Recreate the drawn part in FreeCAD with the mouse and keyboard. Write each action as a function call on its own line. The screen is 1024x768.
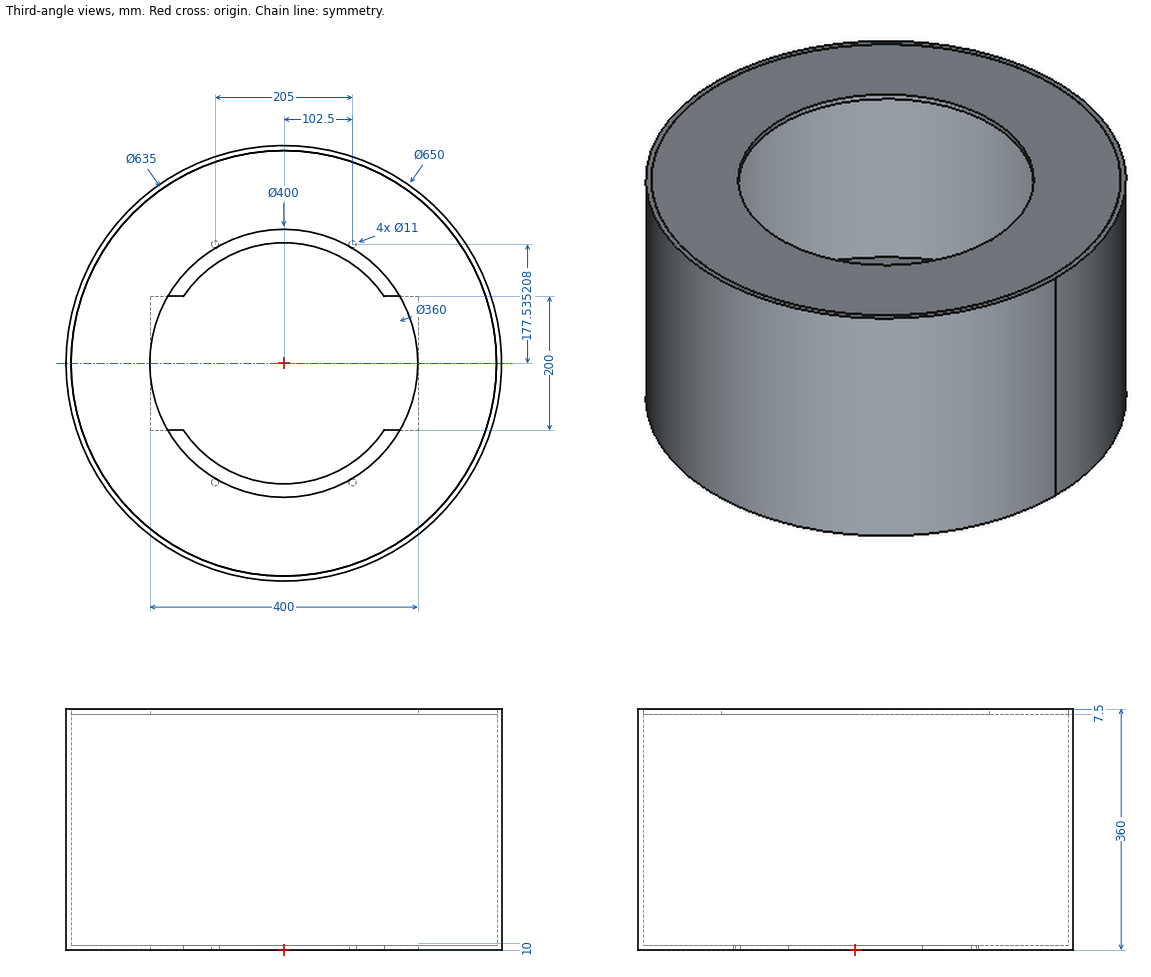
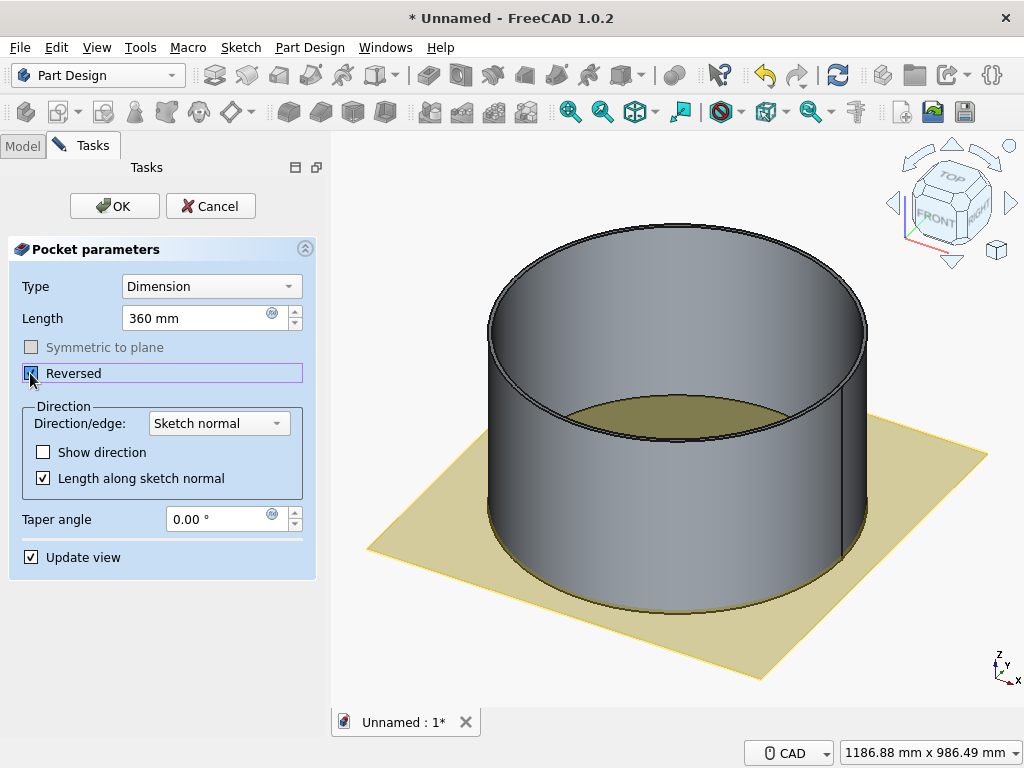
click(115, 206)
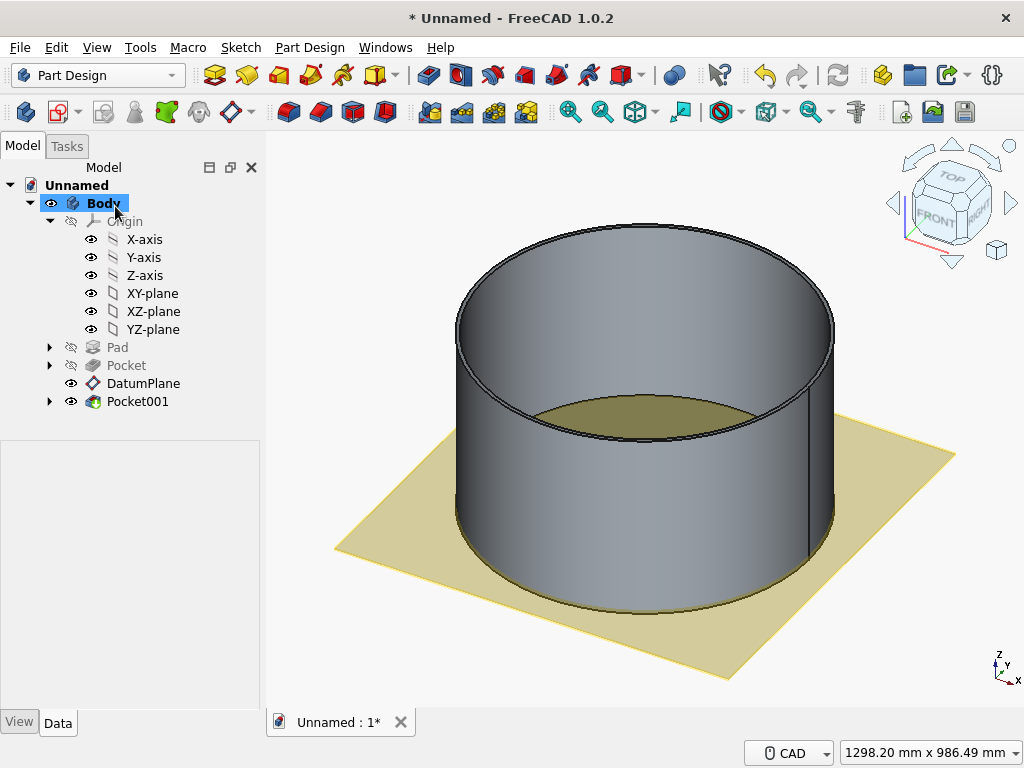
click(116, 383)
key(space)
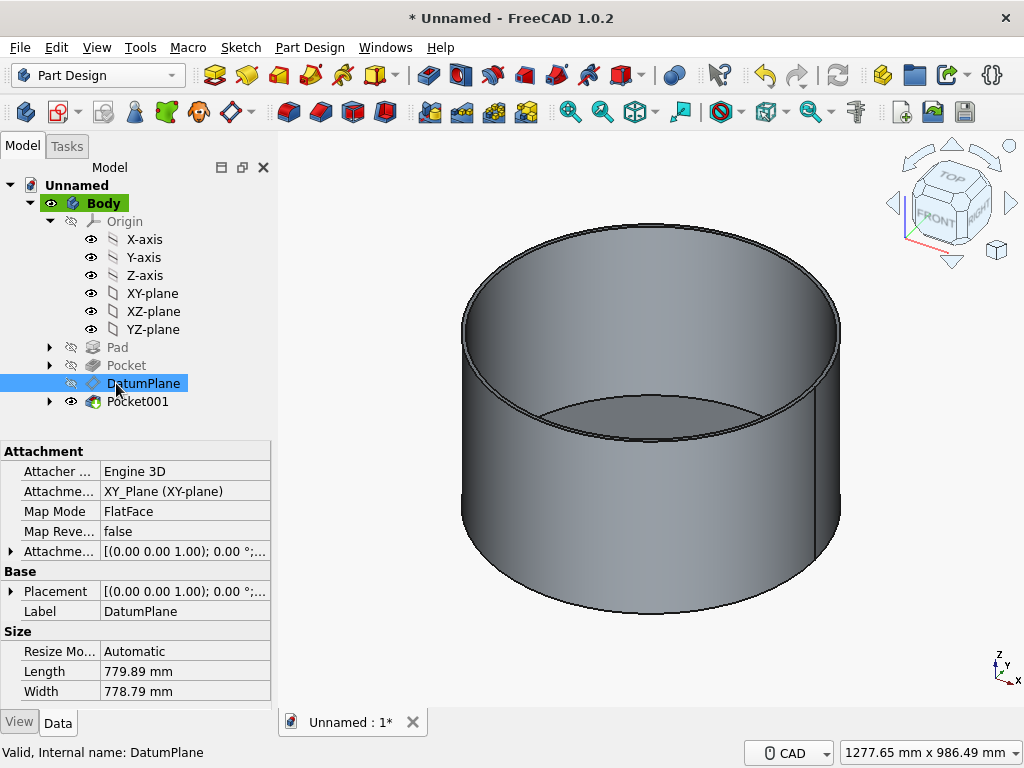
click(318, 667)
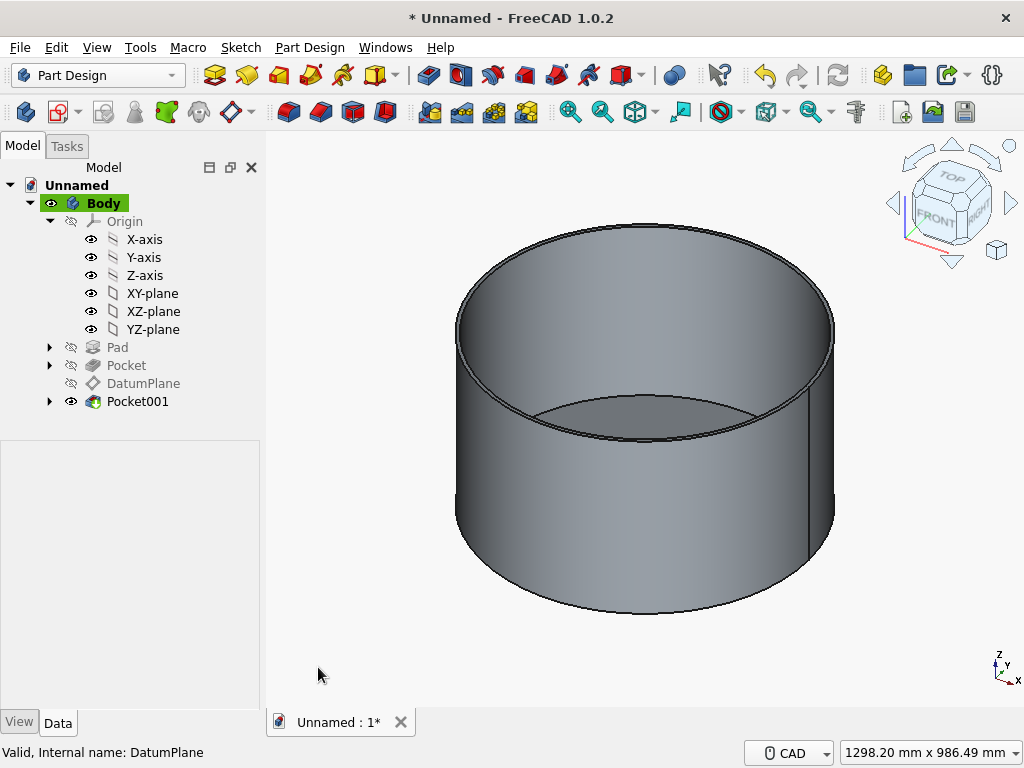
click(58, 112)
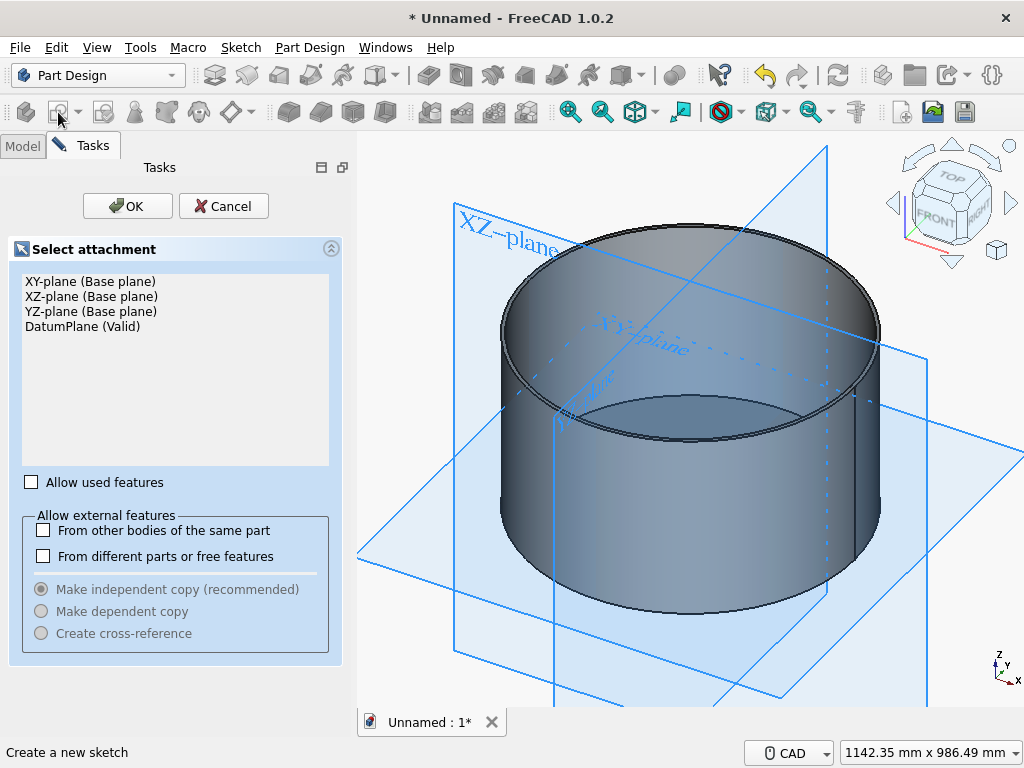
click(82, 282)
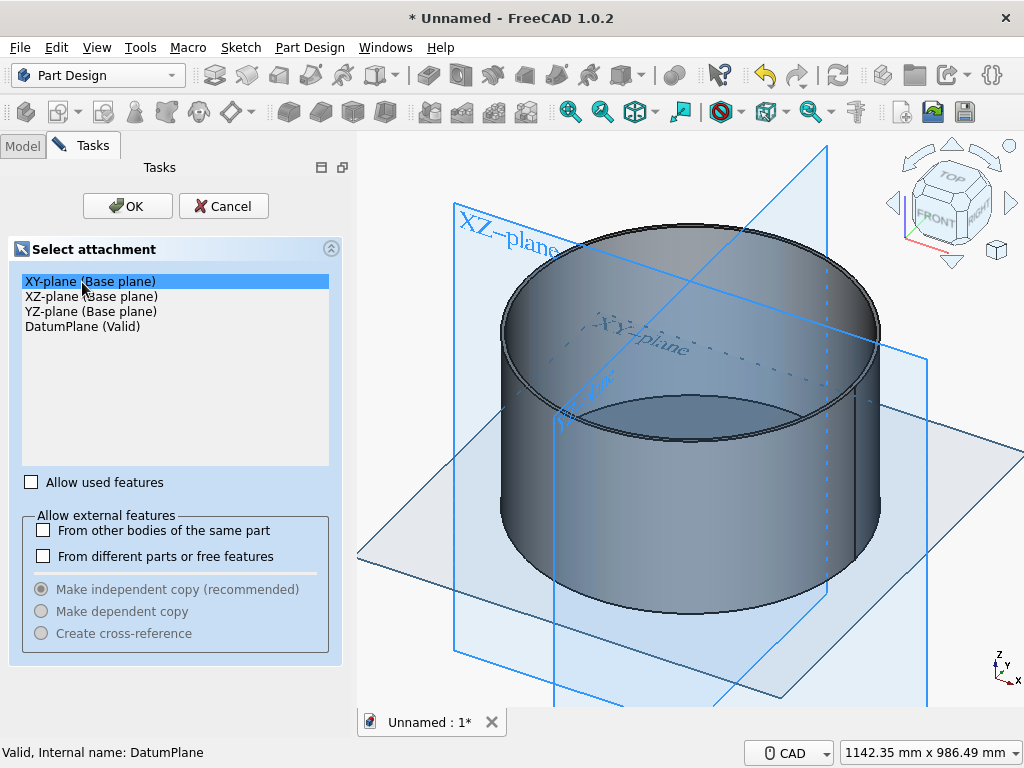
click(128, 206)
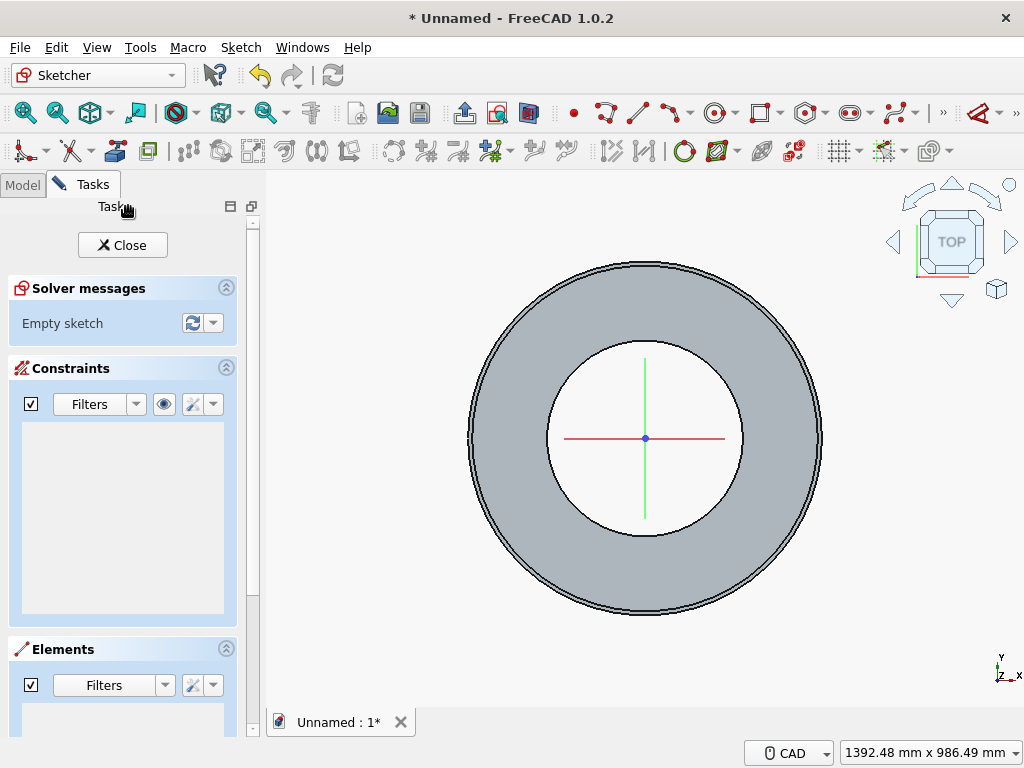
click(530, 114)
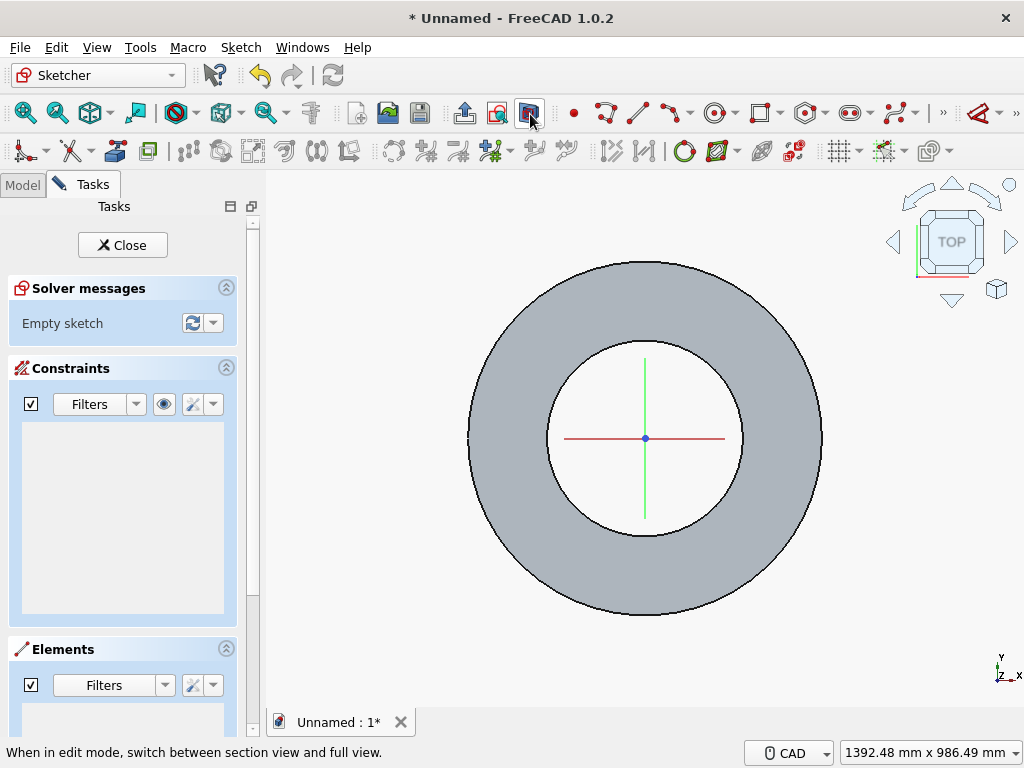
scroll(728, 438, up, 3)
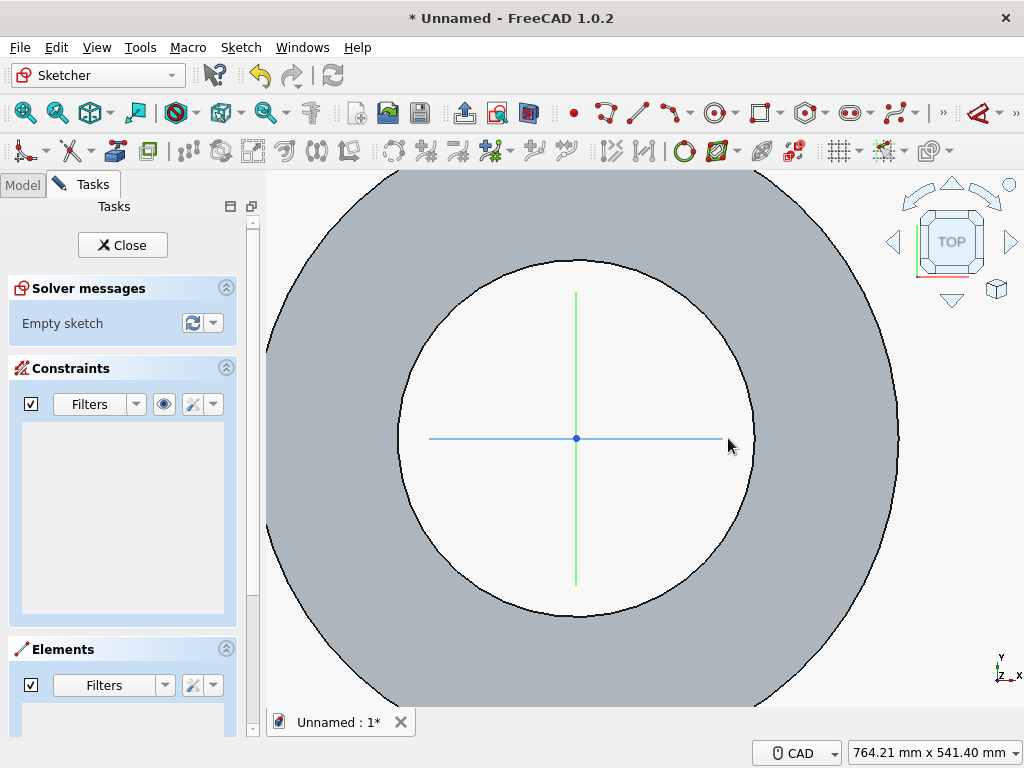
key(g)
key(v)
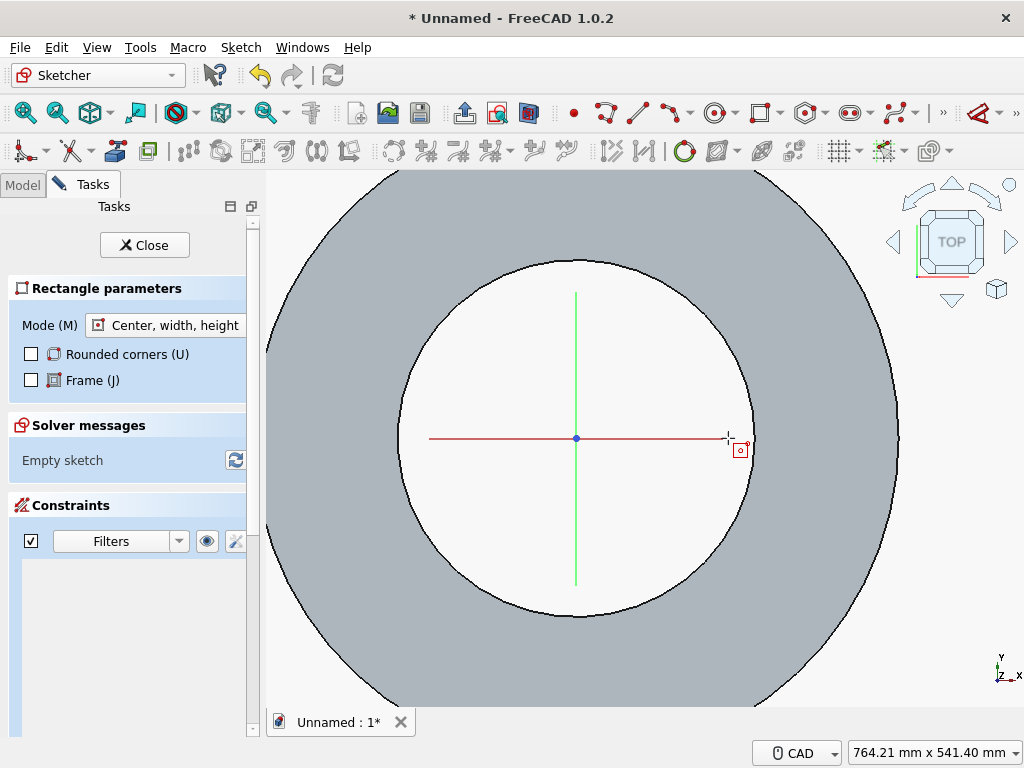
click(576, 438)
click(775, 339)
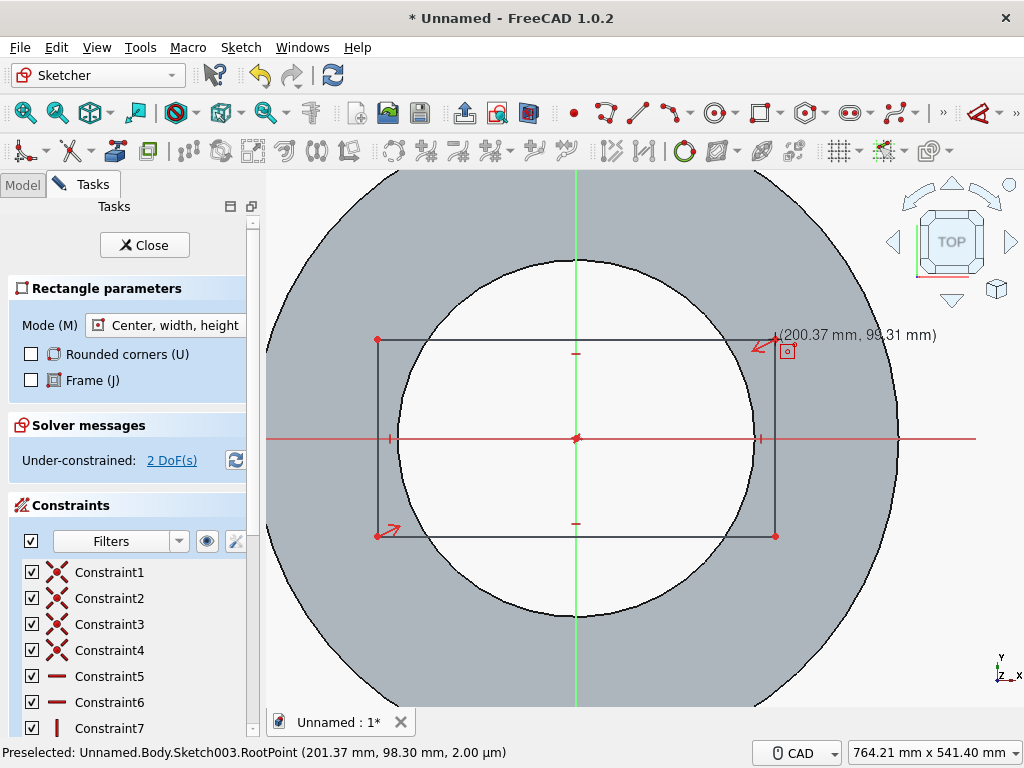
click(716, 114)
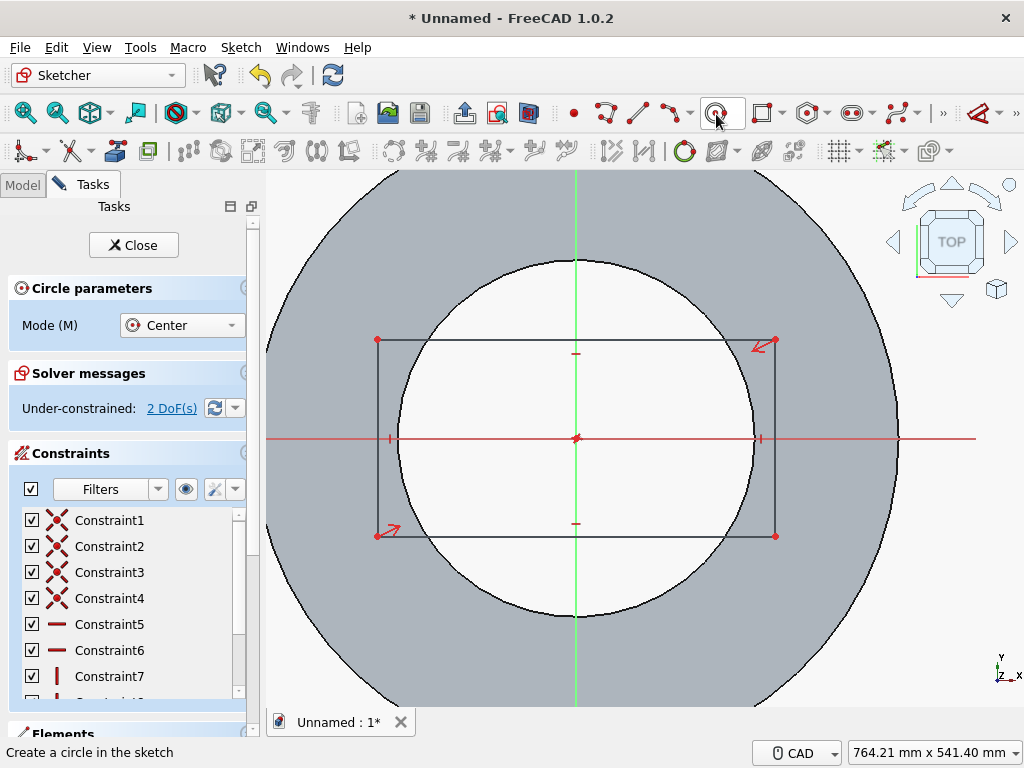
scroll(678, 262, up, 8)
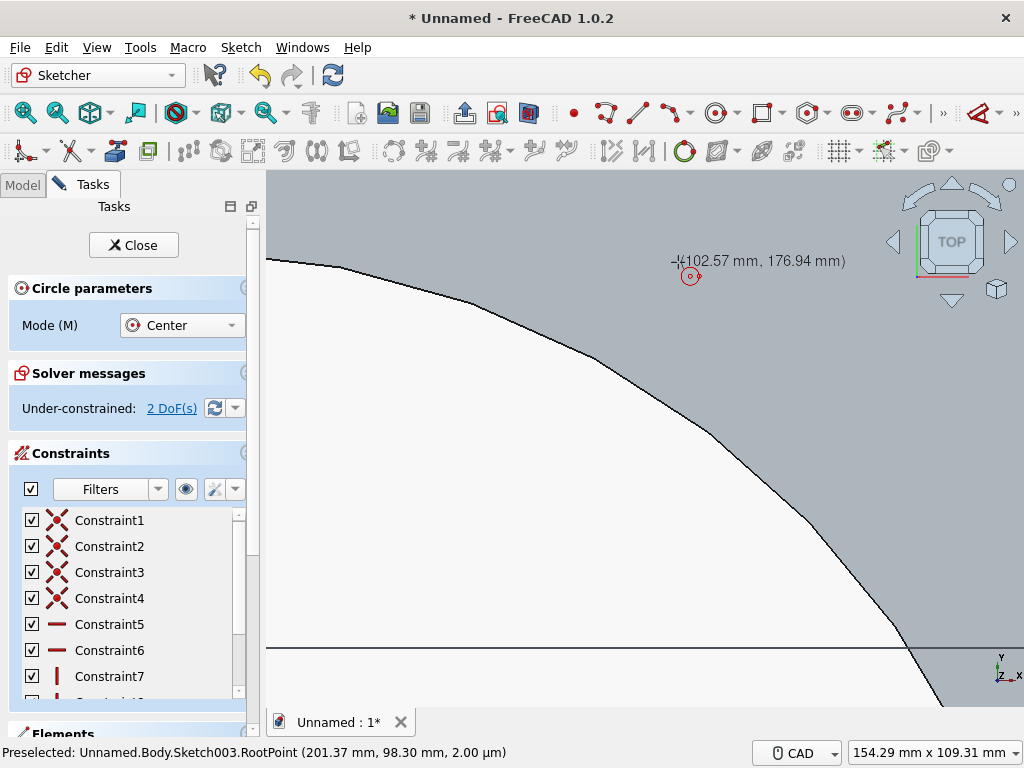
scroll(679, 262, down, 8)